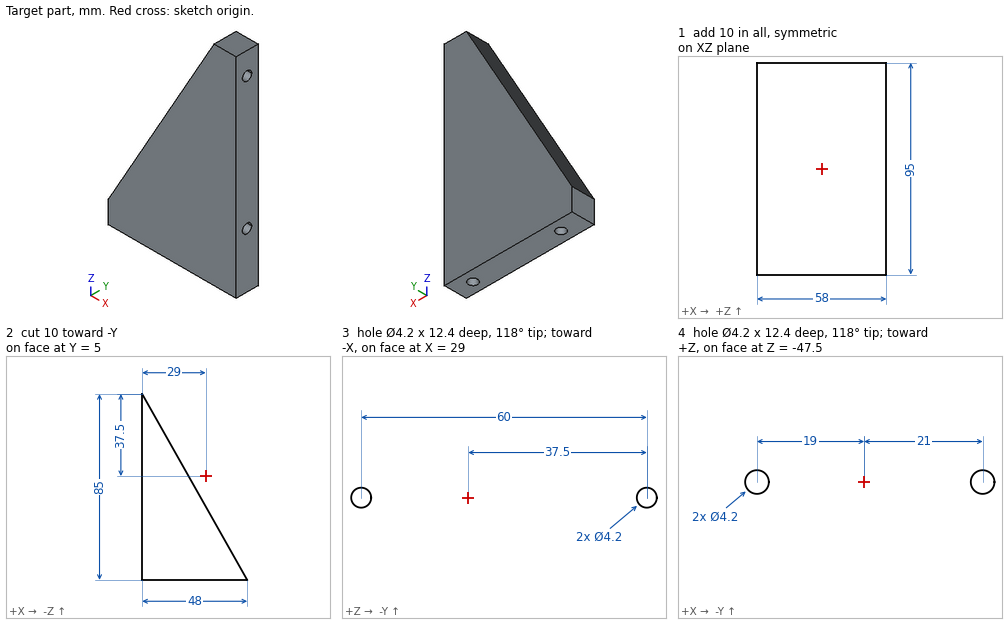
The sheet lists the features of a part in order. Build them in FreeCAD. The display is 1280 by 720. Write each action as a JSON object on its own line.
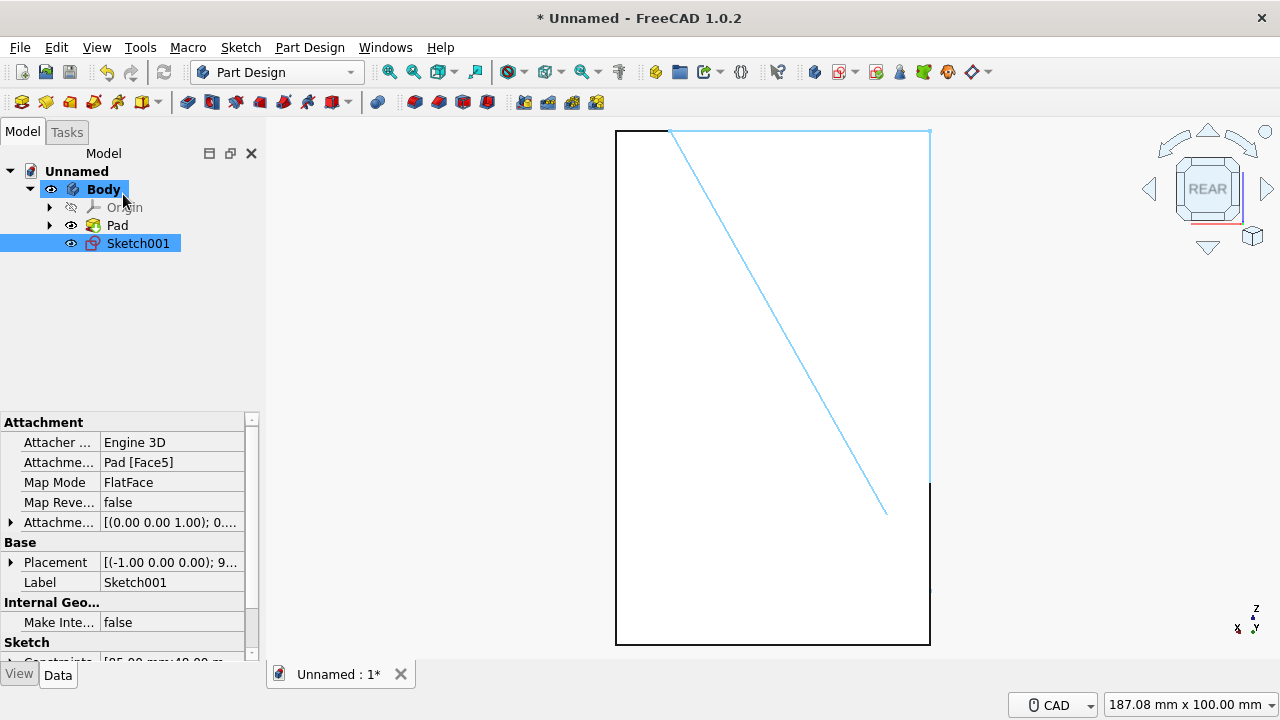
{"action": "left_click", "coordinate": [188, 102]}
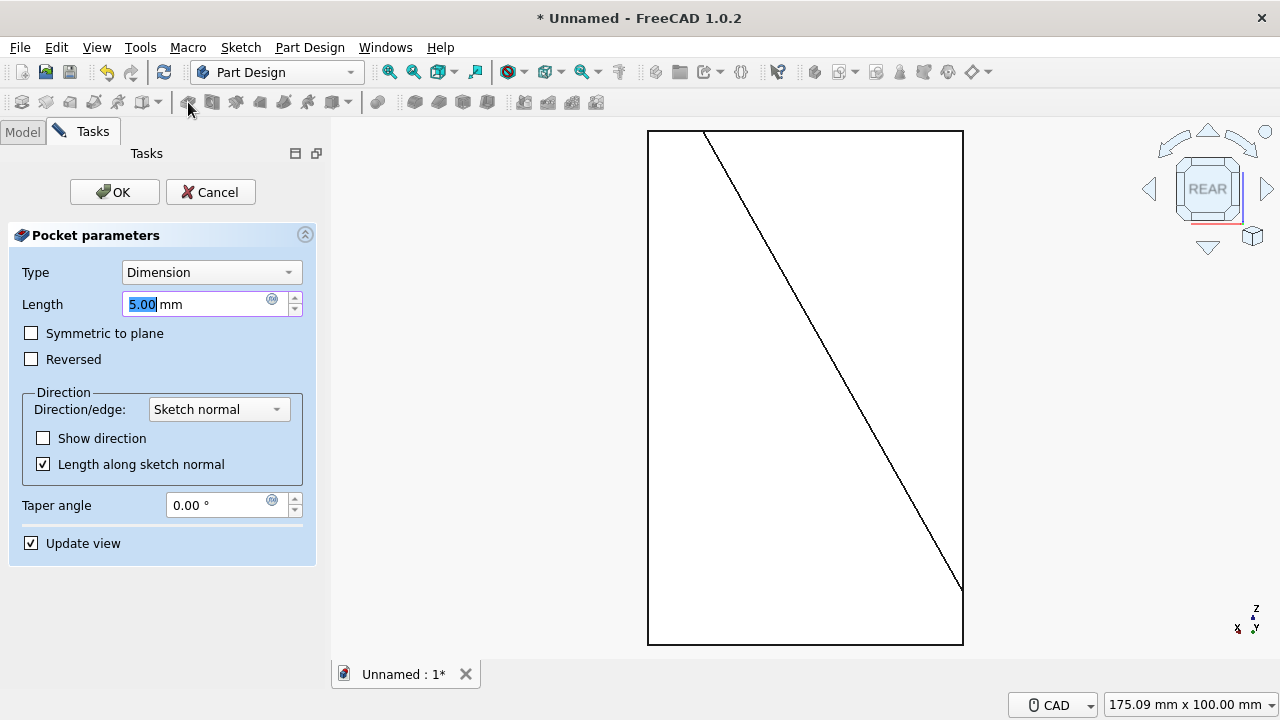
{"action": "type", "text": "10"}
{"action": "key", "text": "Tab"}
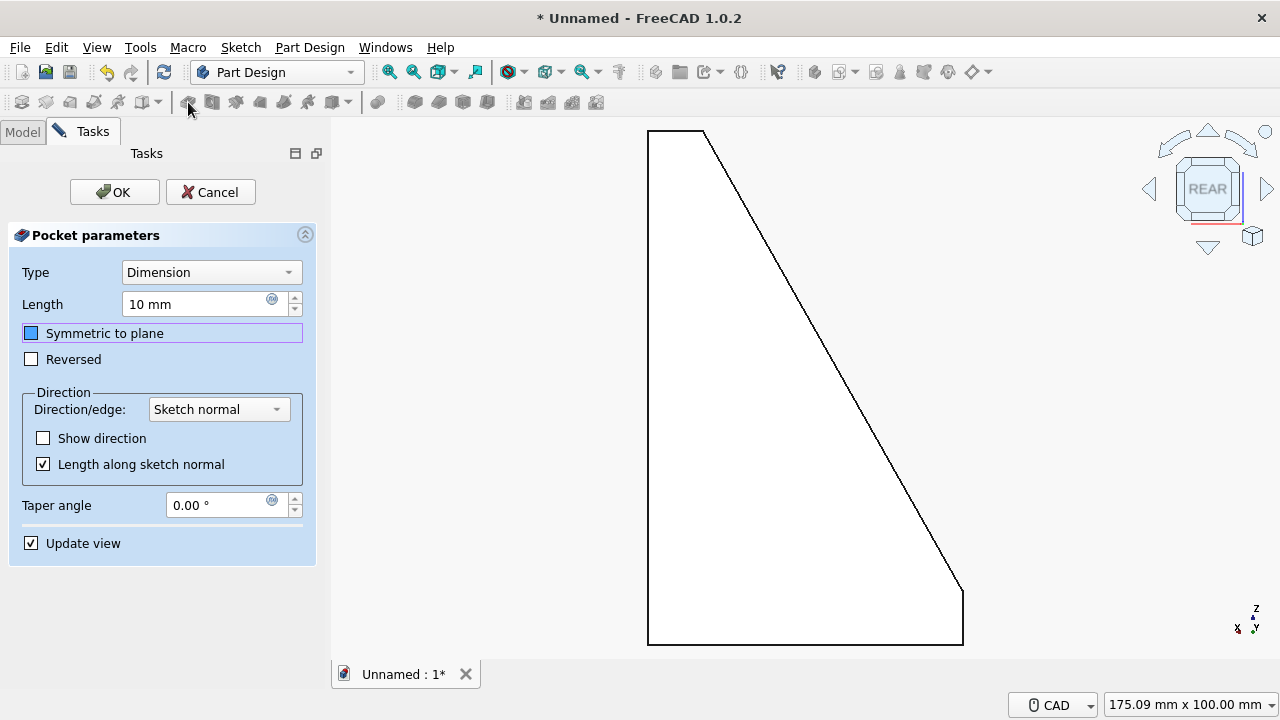
{"action": "left_click", "coordinate": [115, 192]}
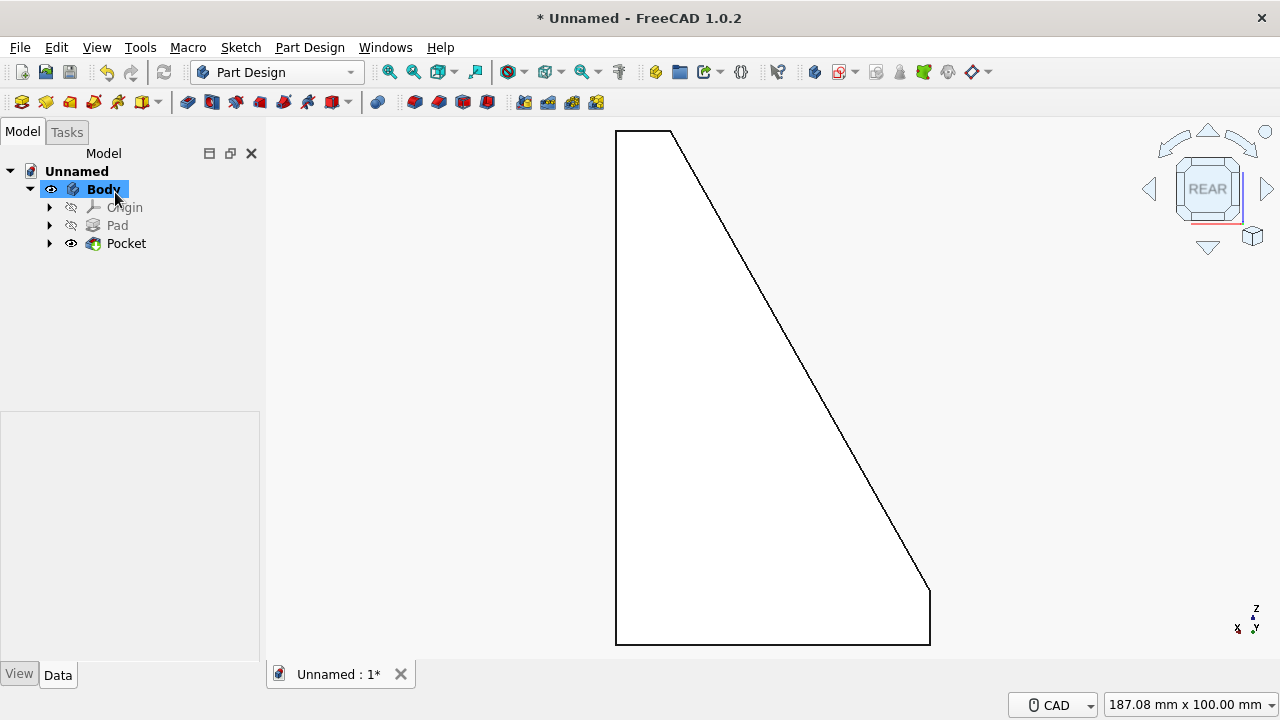
{"action": "key", "text": "0"}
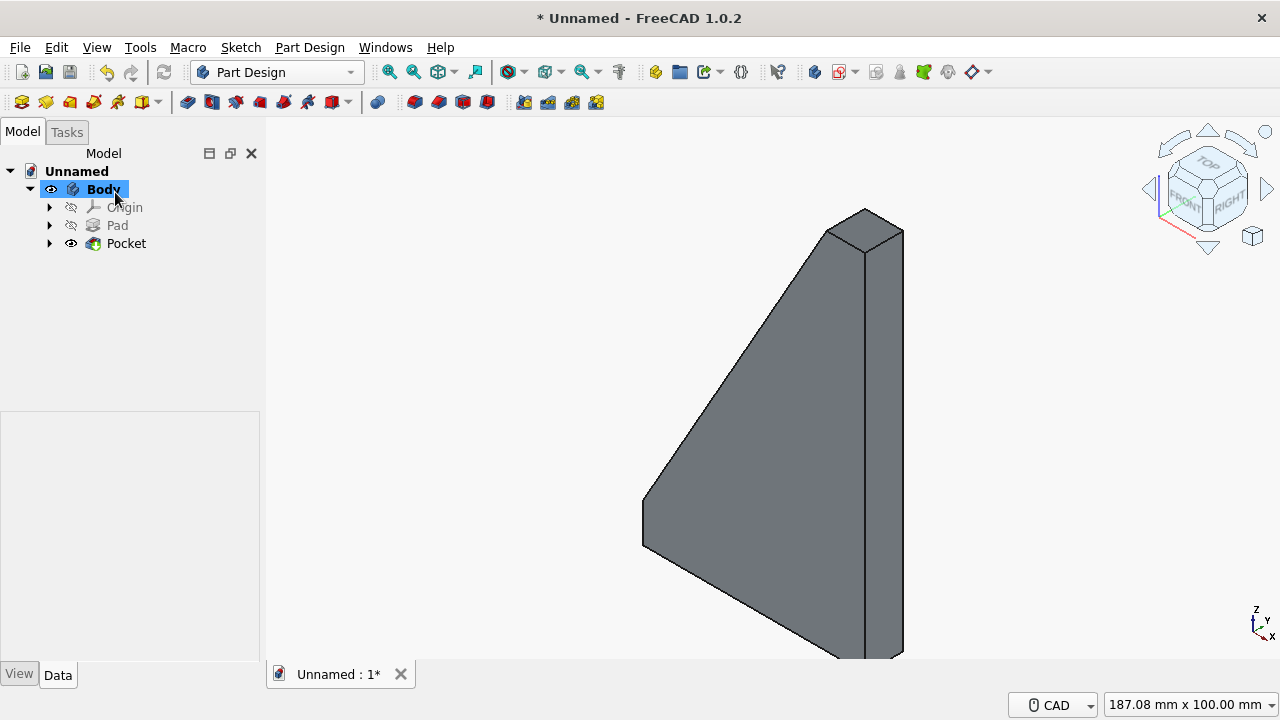
{"action": "left_click", "coordinate": [390, 72]}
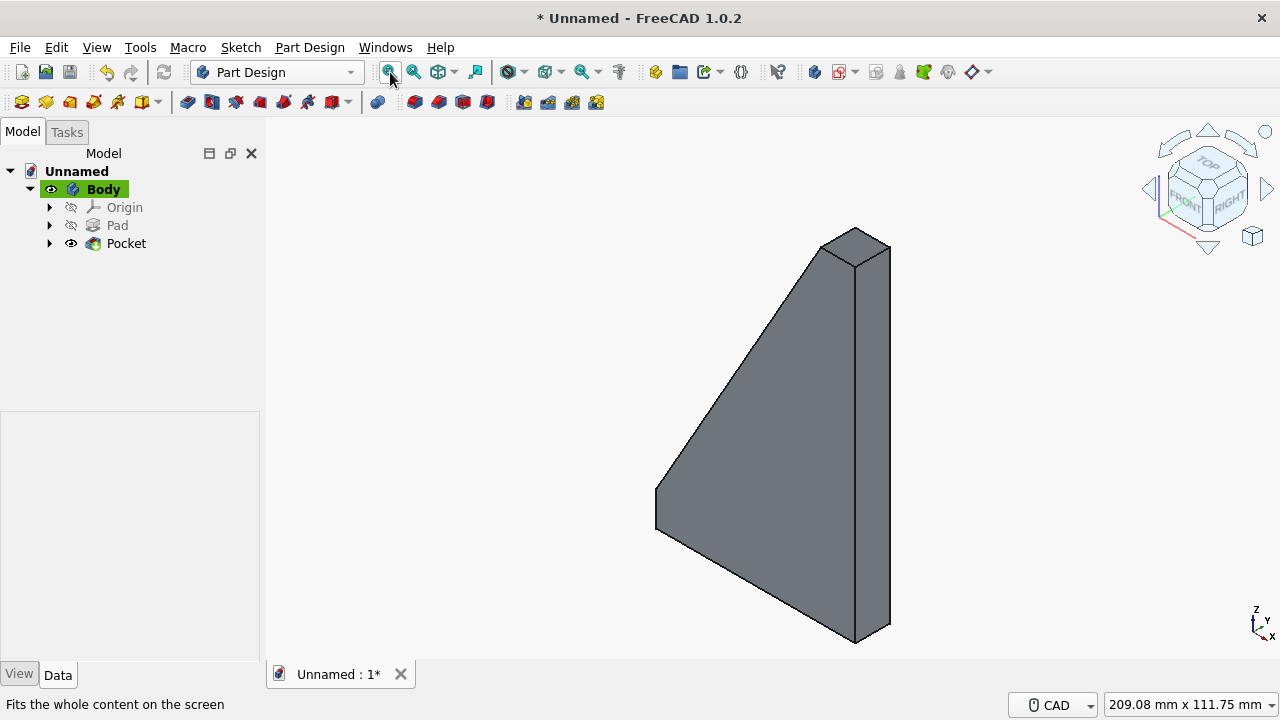
{"action": "left_click", "coordinate": [872, 283]}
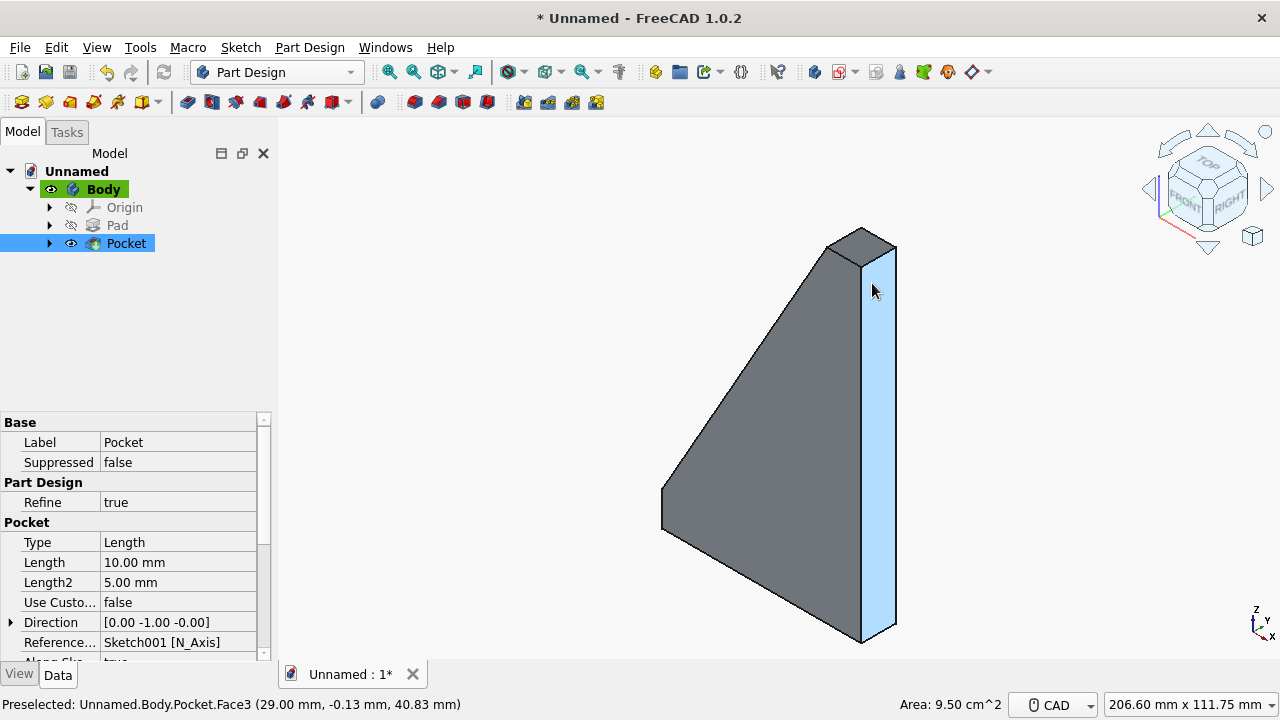
{"action": "left_click", "coordinate": [840, 72]}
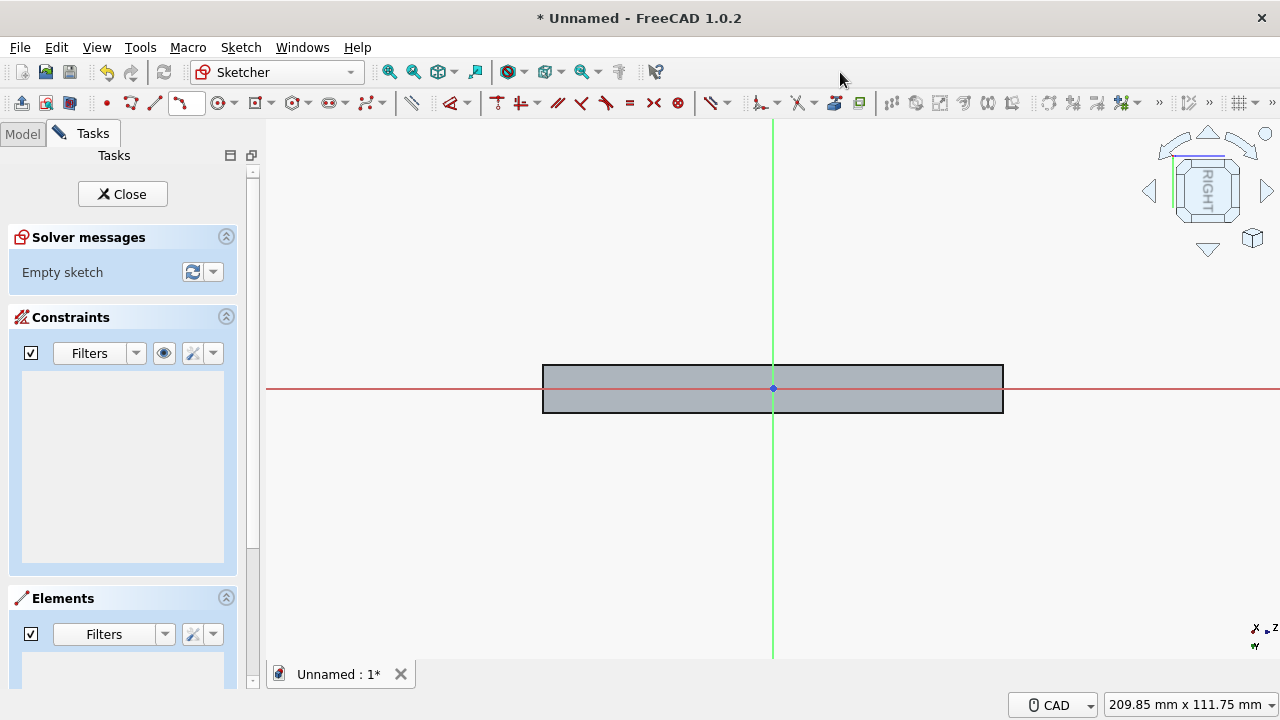
{"action": "scroll", "coordinate": [937, 389], "scroll_direction": "up", "scroll_amount": 3}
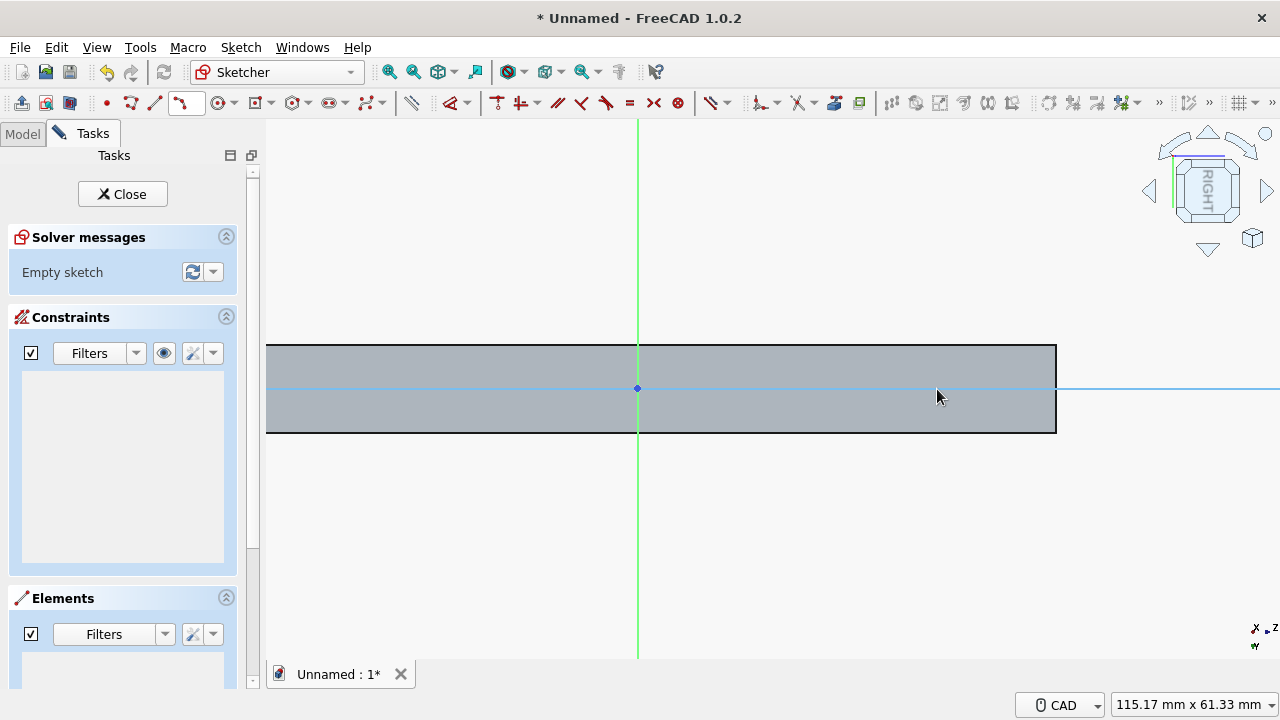
{"action": "left_click", "coordinate": [218, 104]}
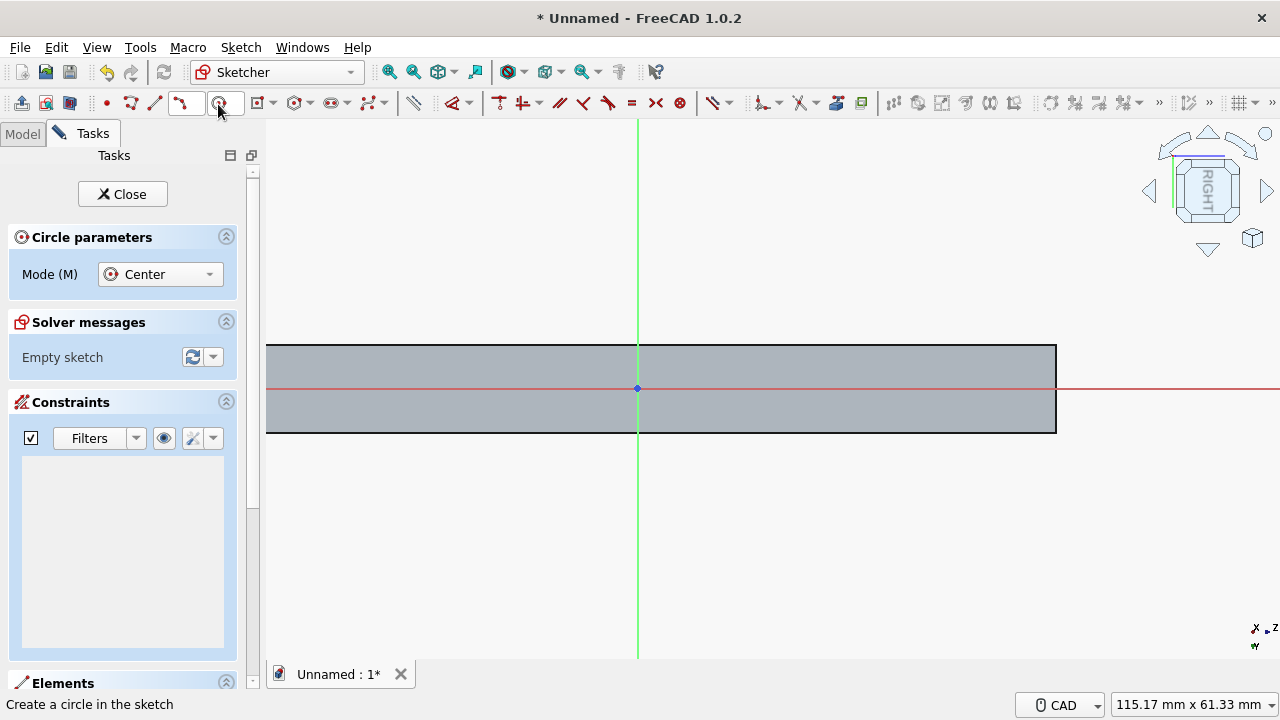
{"action": "scroll", "coordinate": [968, 389], "scroll_direction": "up", "scroll_amount": 2}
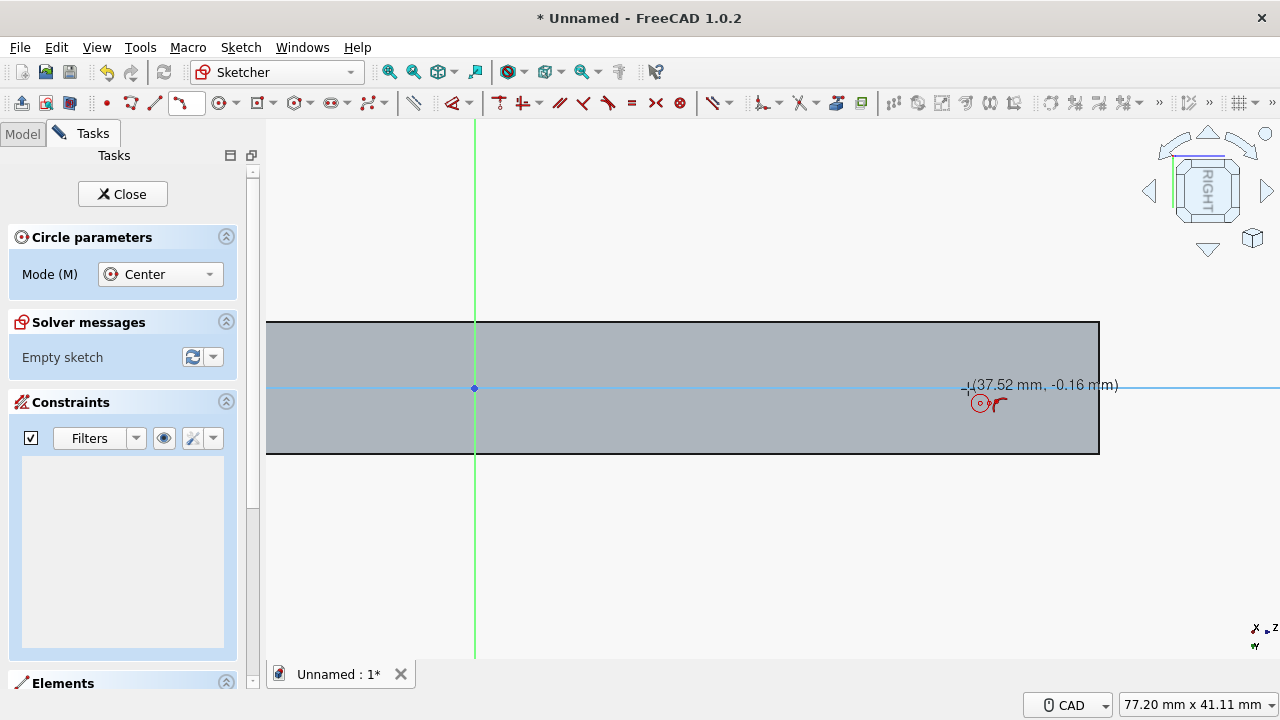
{"action": "left_click", "coordinate": [967, 388]}
{"action": "left_click", "coordinate": [987, 369]}